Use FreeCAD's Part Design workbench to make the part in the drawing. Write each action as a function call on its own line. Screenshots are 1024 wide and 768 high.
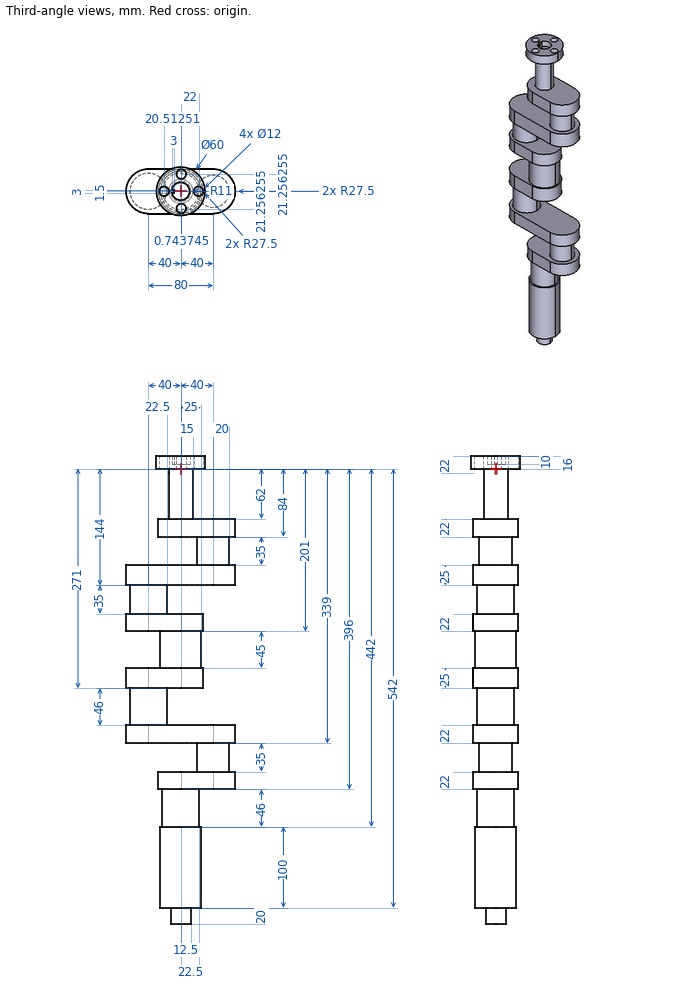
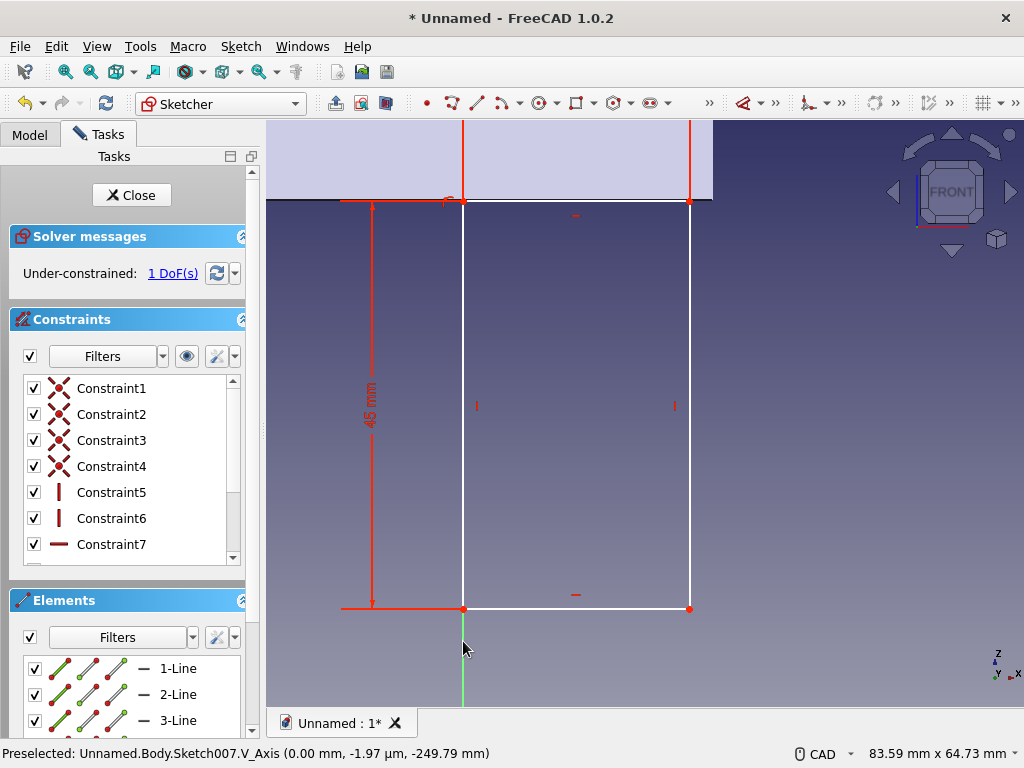
click(742, 104)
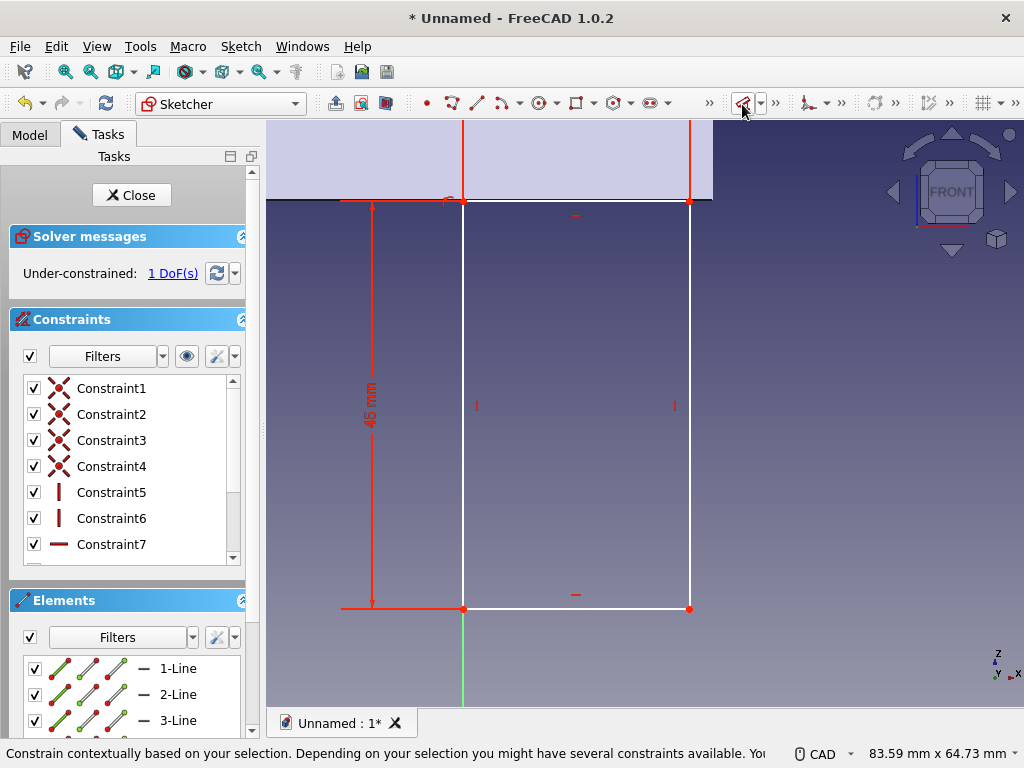
click(463, 201)
click(429, 175)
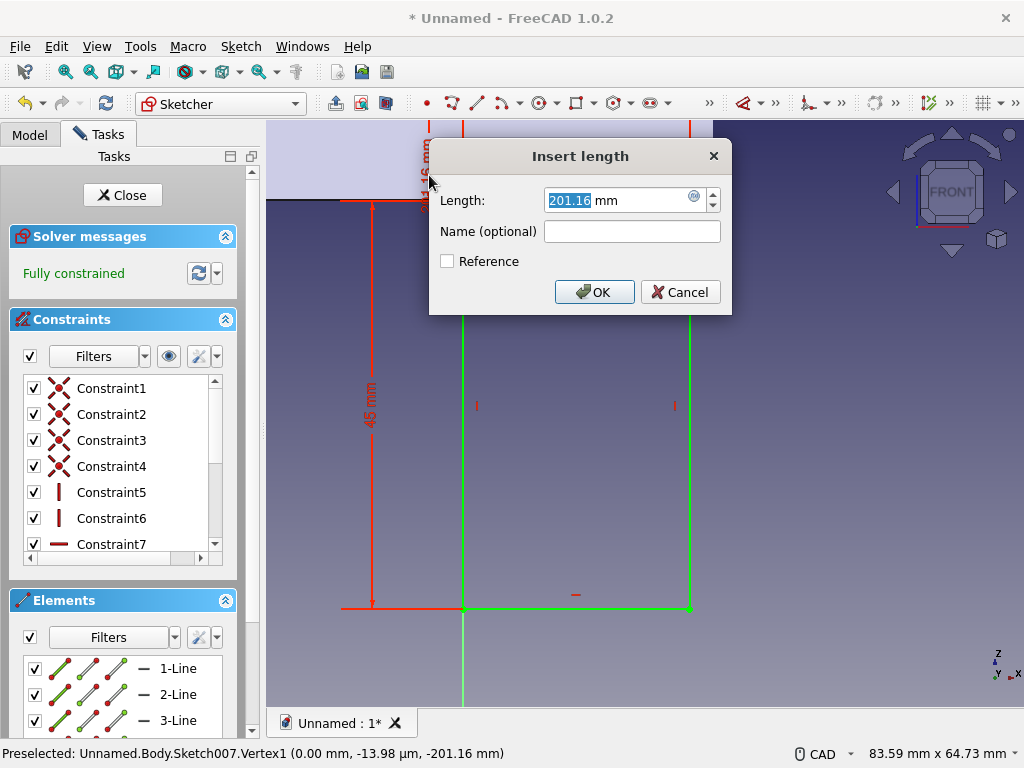
text(201)
key(Return)
key(Escape)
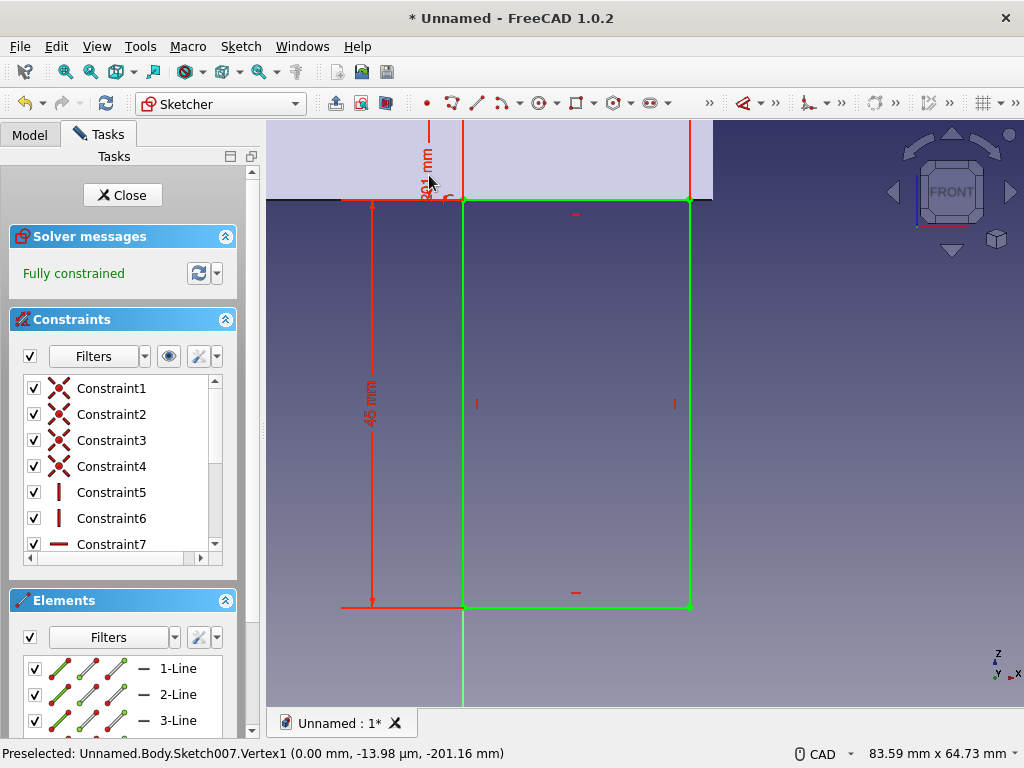
click(123, 195)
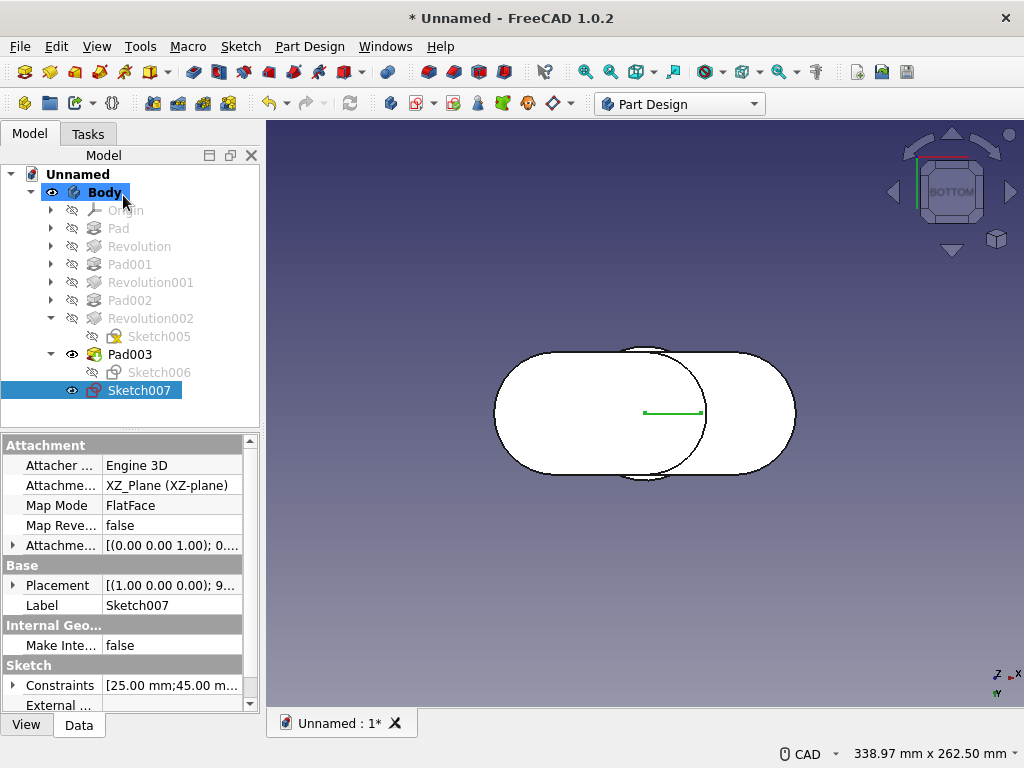
click(50, 72)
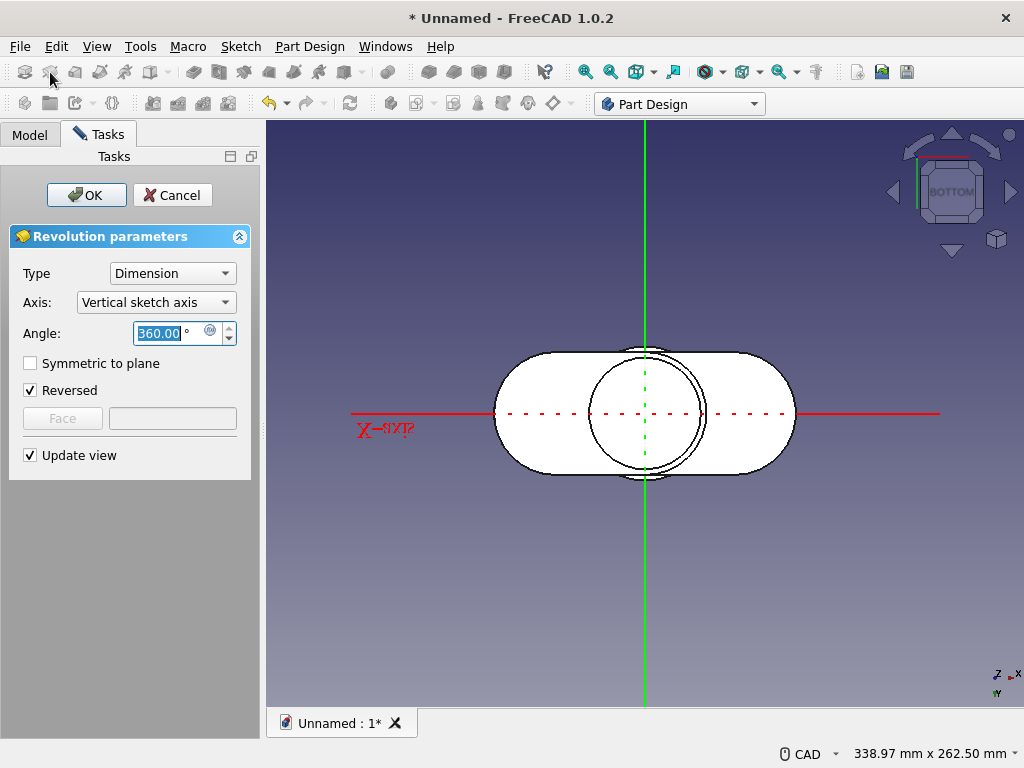
click(87, 195)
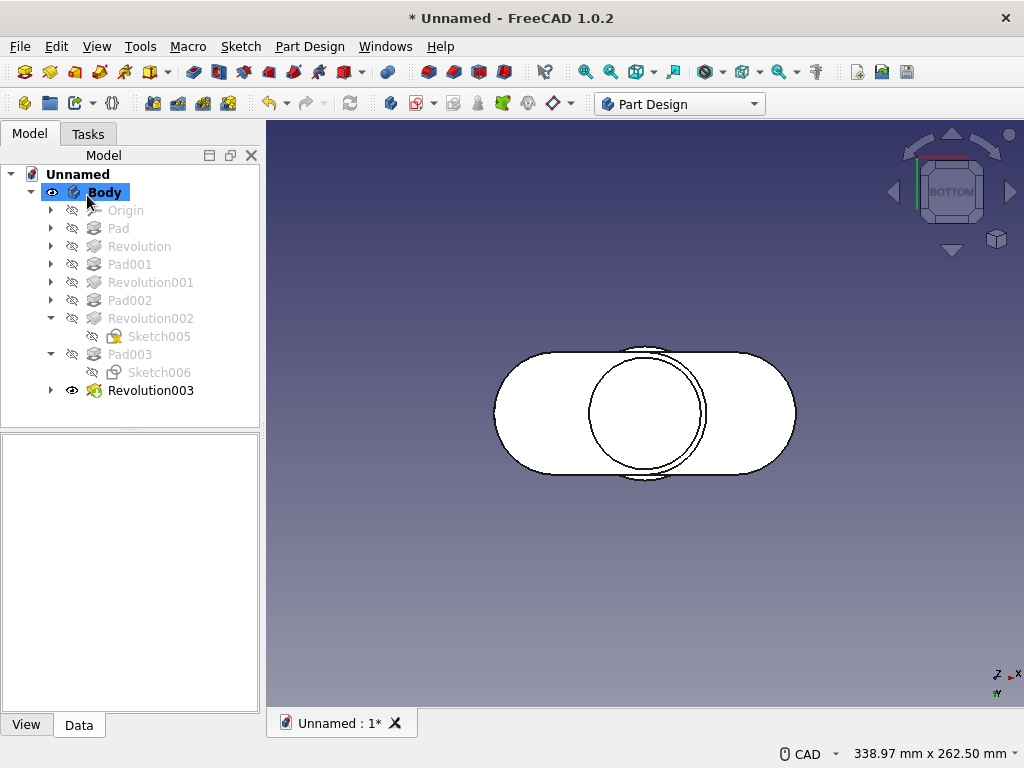
click(586, 72)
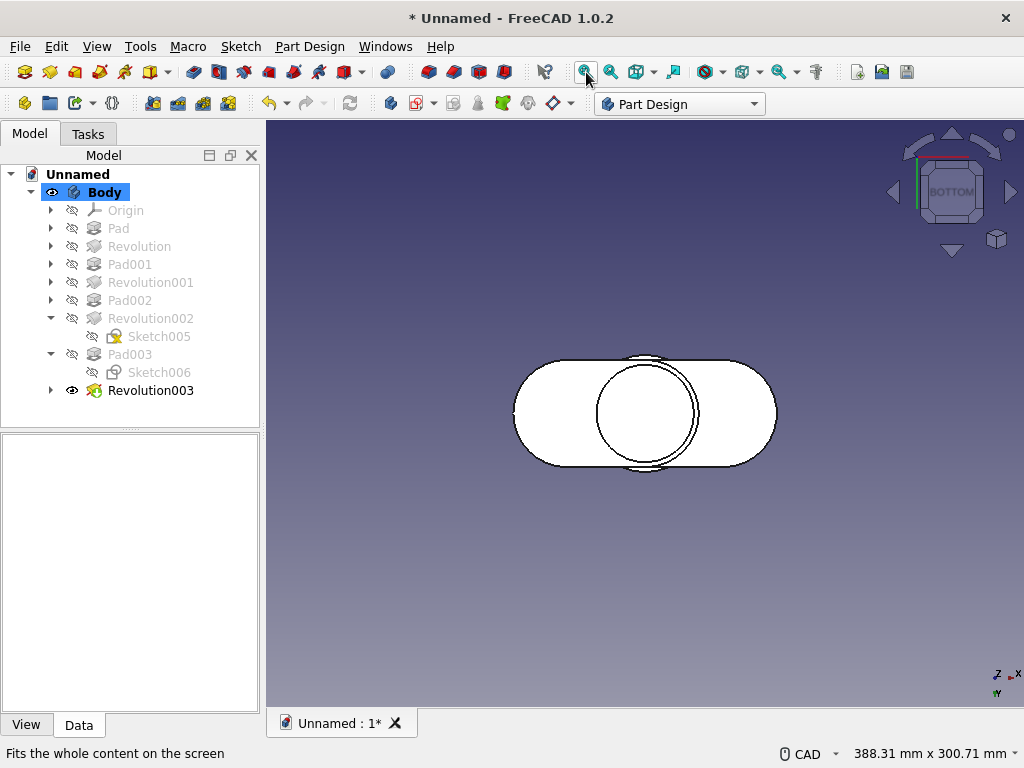
click(645, 412)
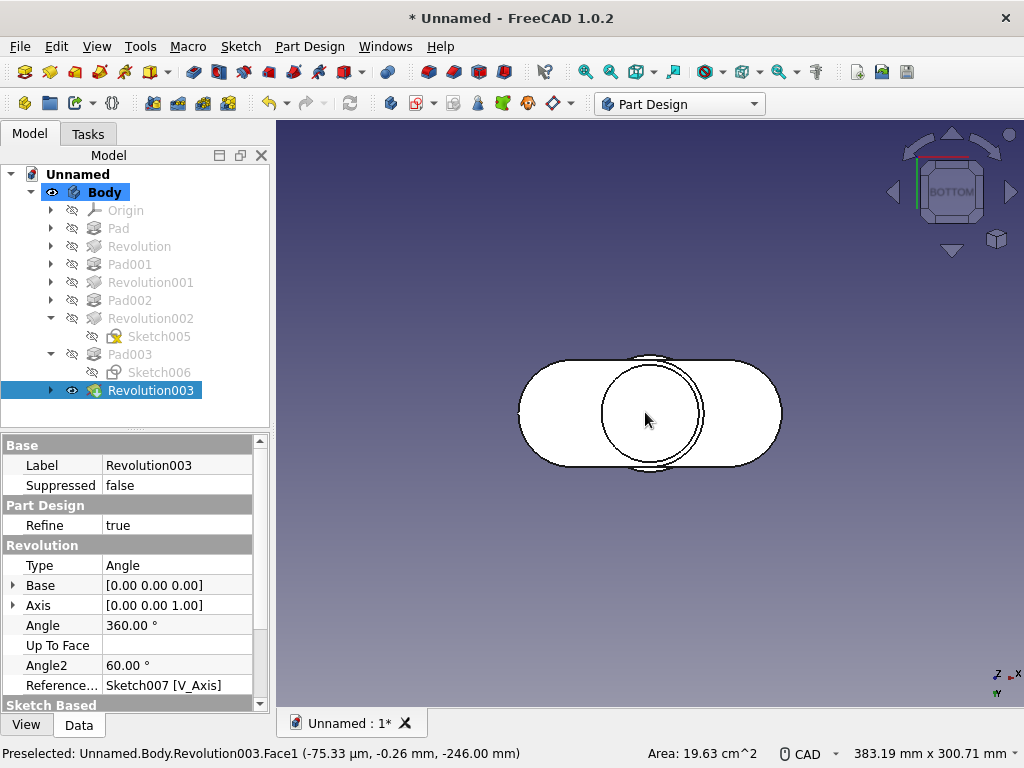
click(416, 104)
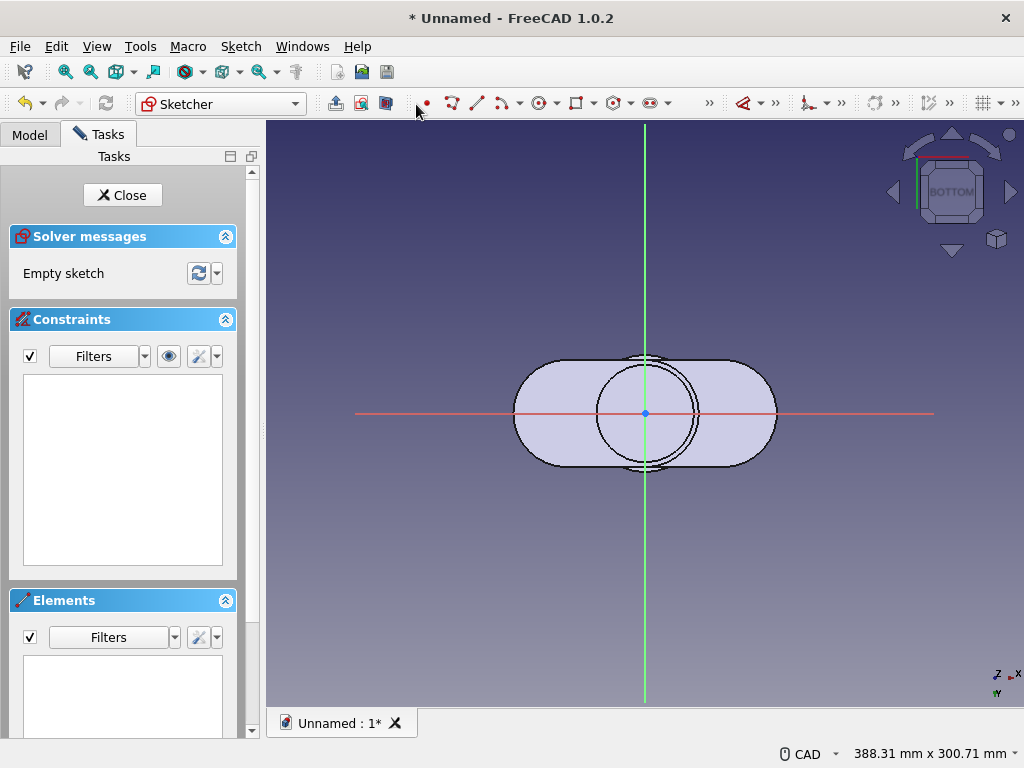
scroll(630, 413, up, 4)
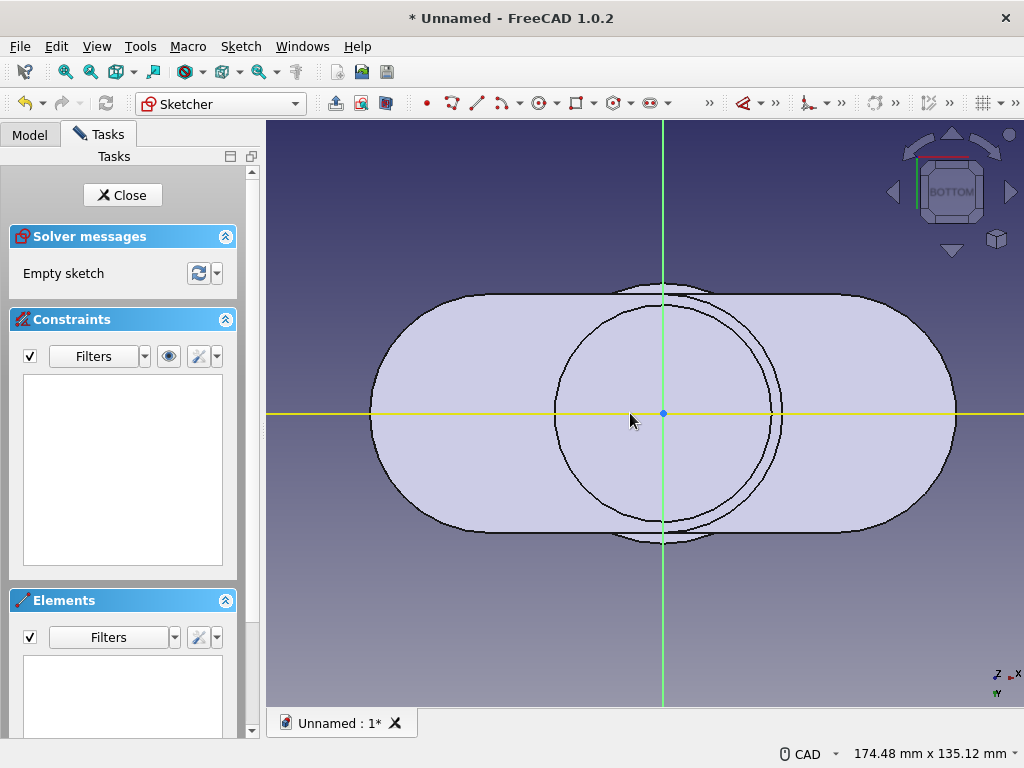
click(650, 104)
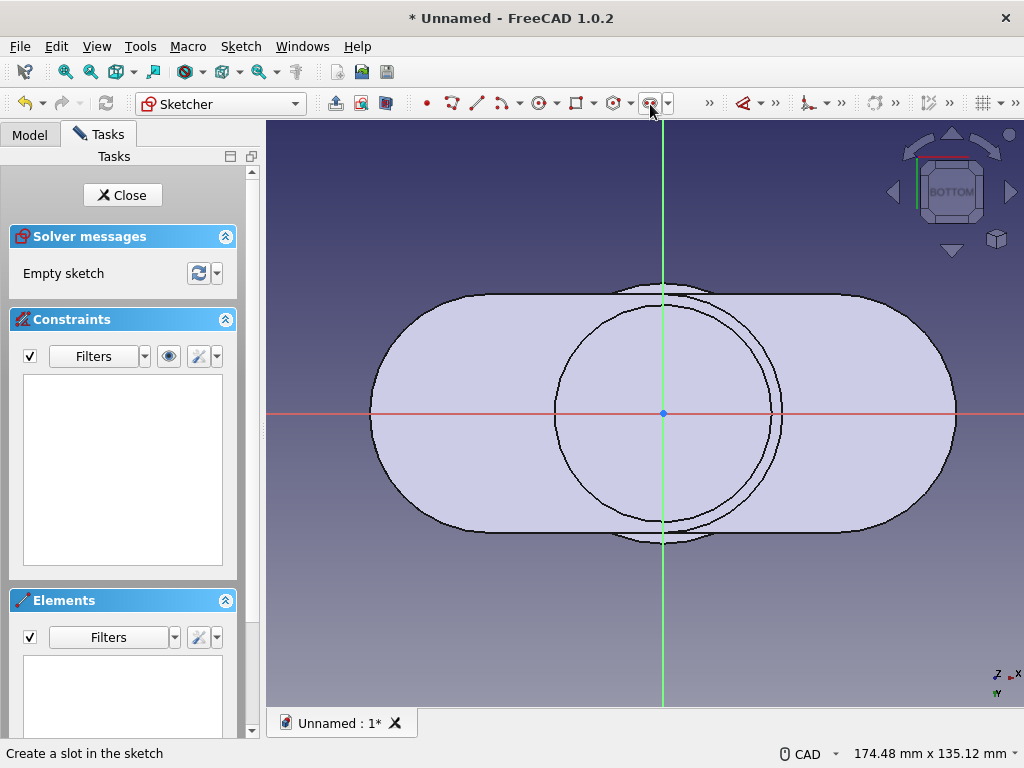
click(663, 413)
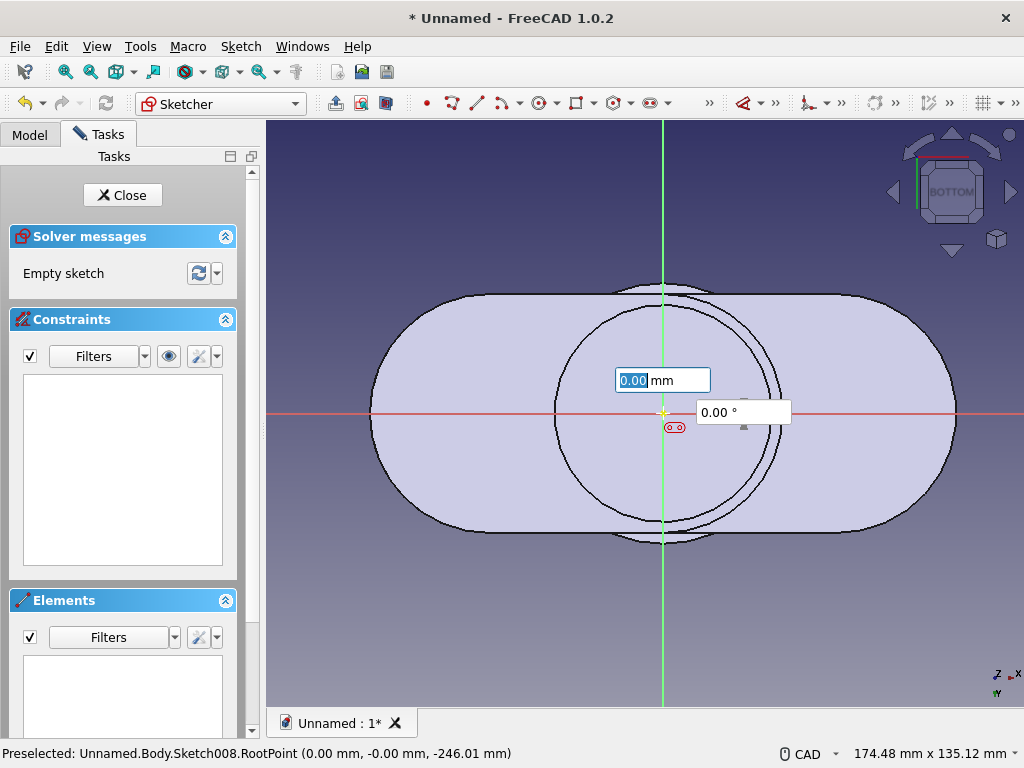
click(489, 404)